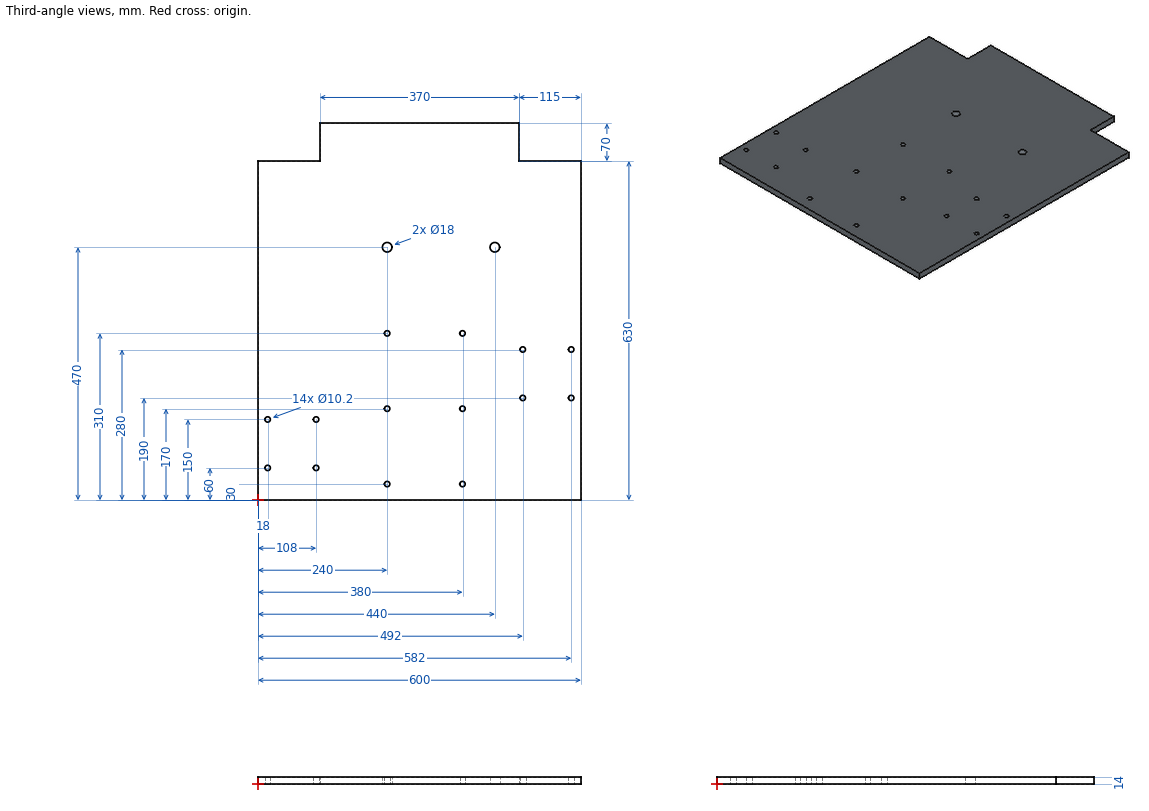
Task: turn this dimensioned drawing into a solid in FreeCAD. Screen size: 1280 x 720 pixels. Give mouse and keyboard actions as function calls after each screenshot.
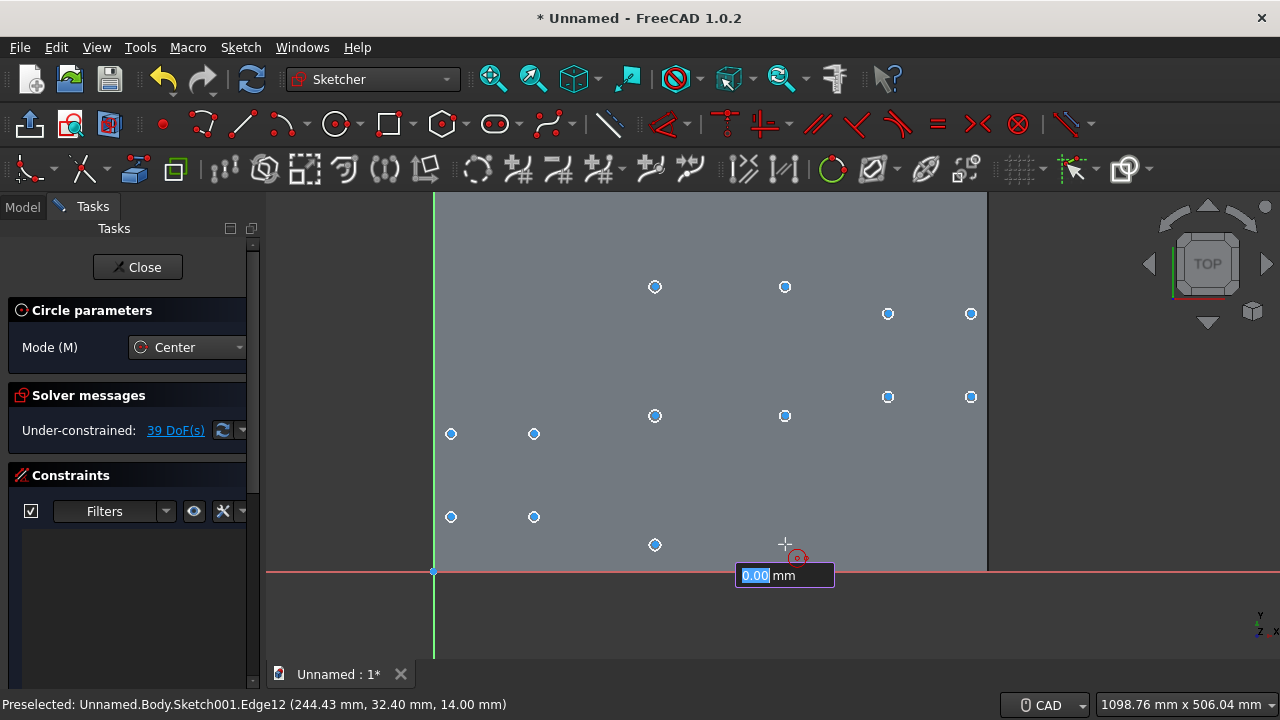
scroll(788, 541, up, 7)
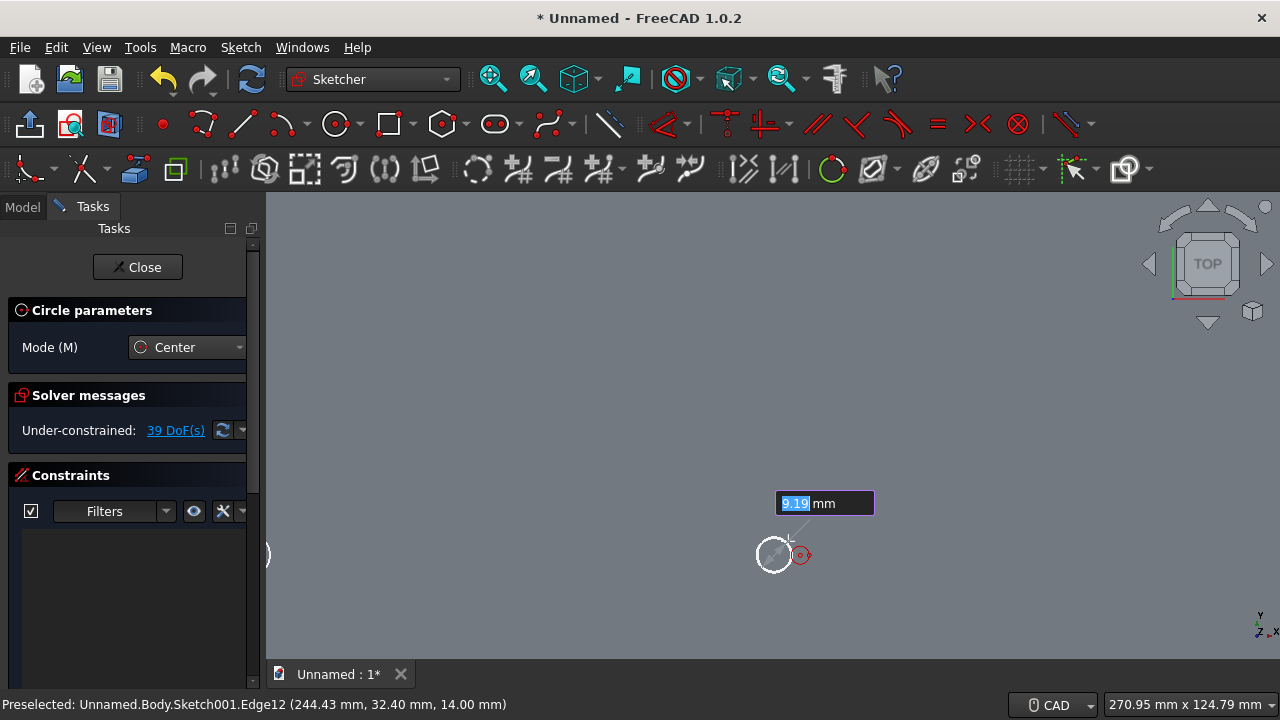
click(786, 537)
key(Escape)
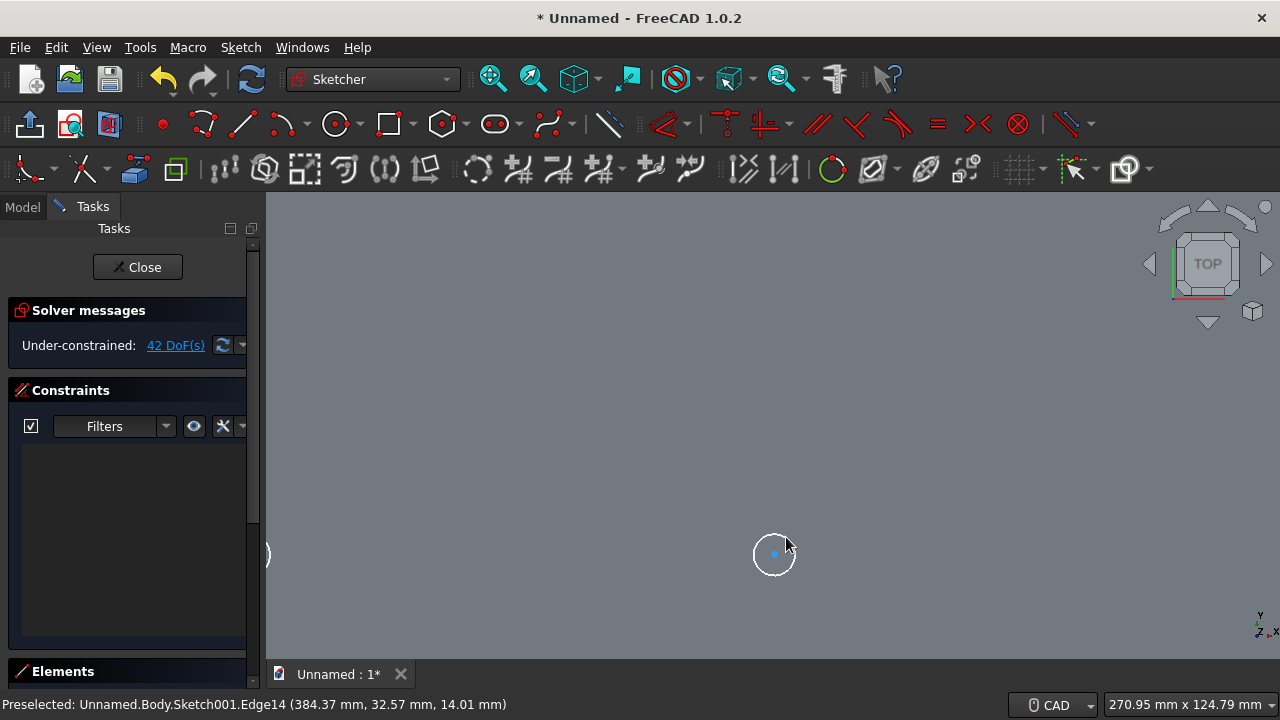
scroll(788, 541, down, 7)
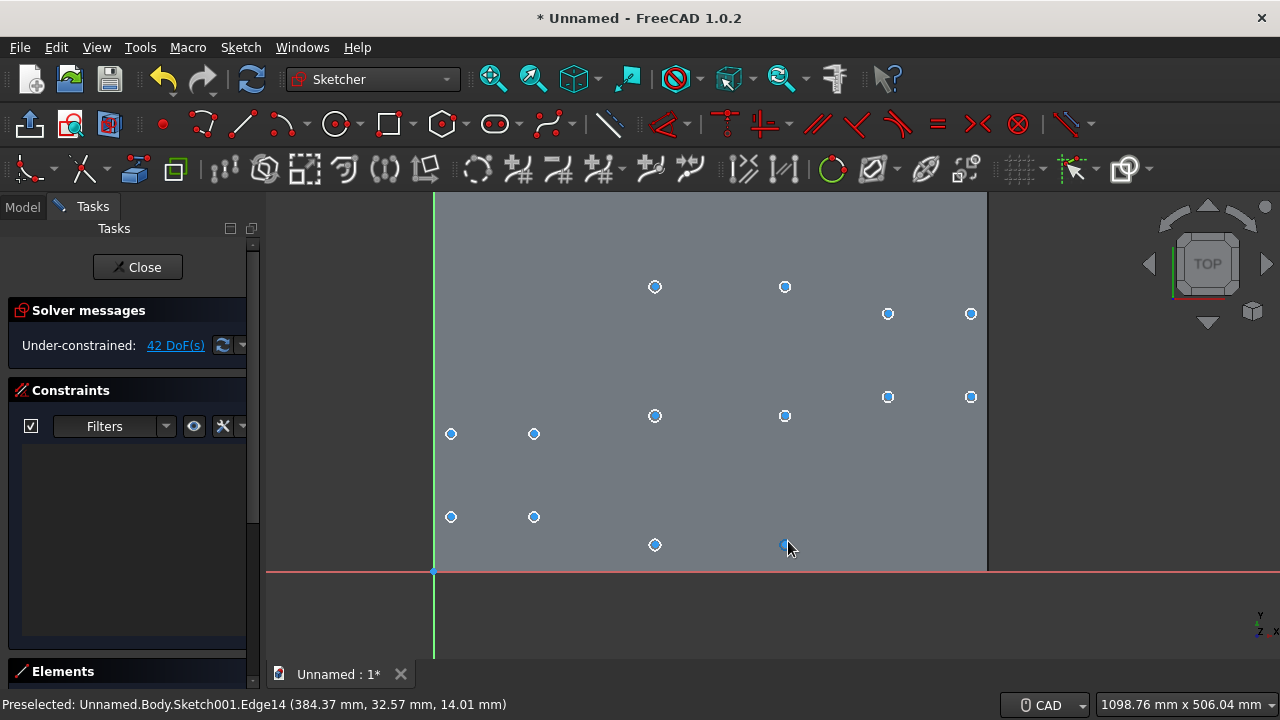
scroll(454, 431, up, 6)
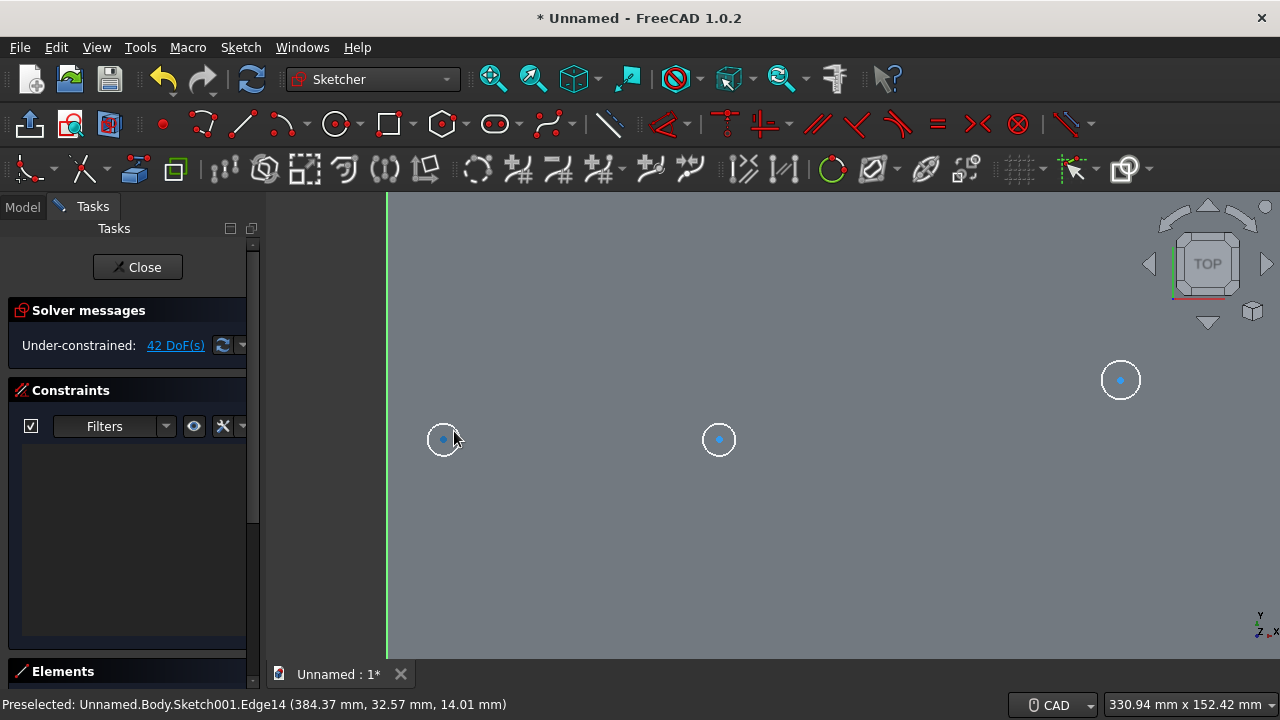
click(455, 428)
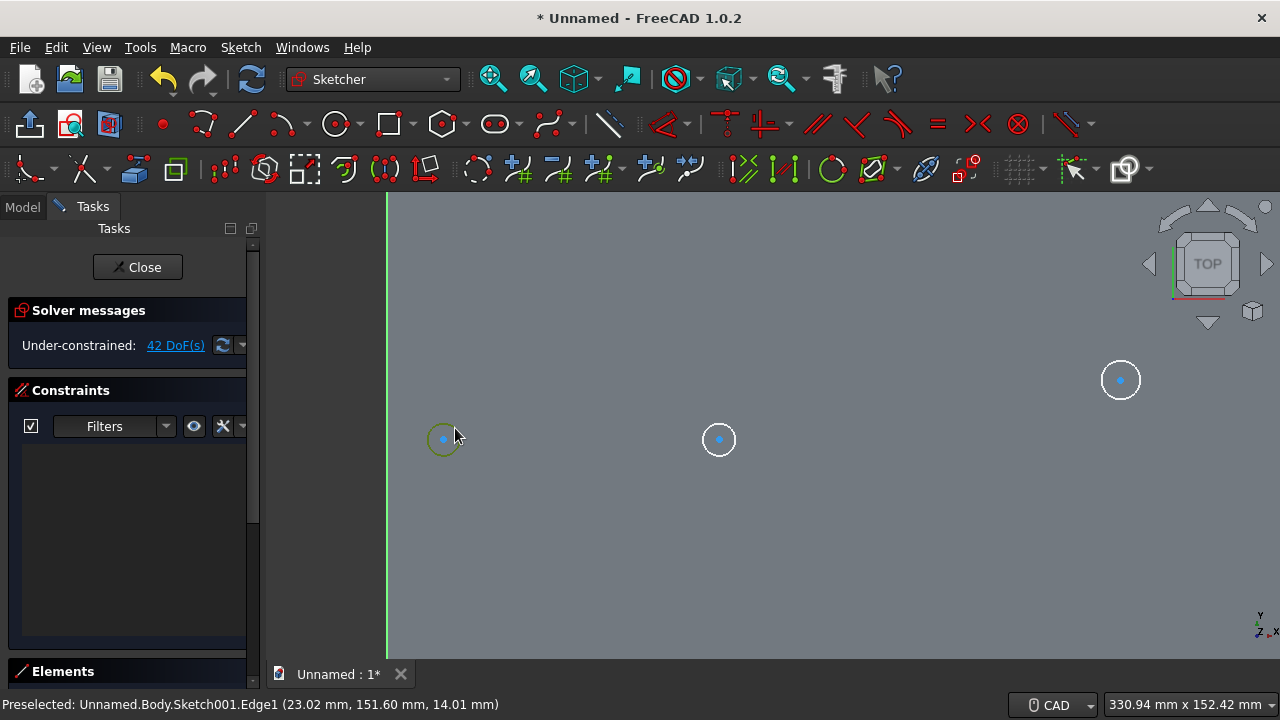
click(731, 428)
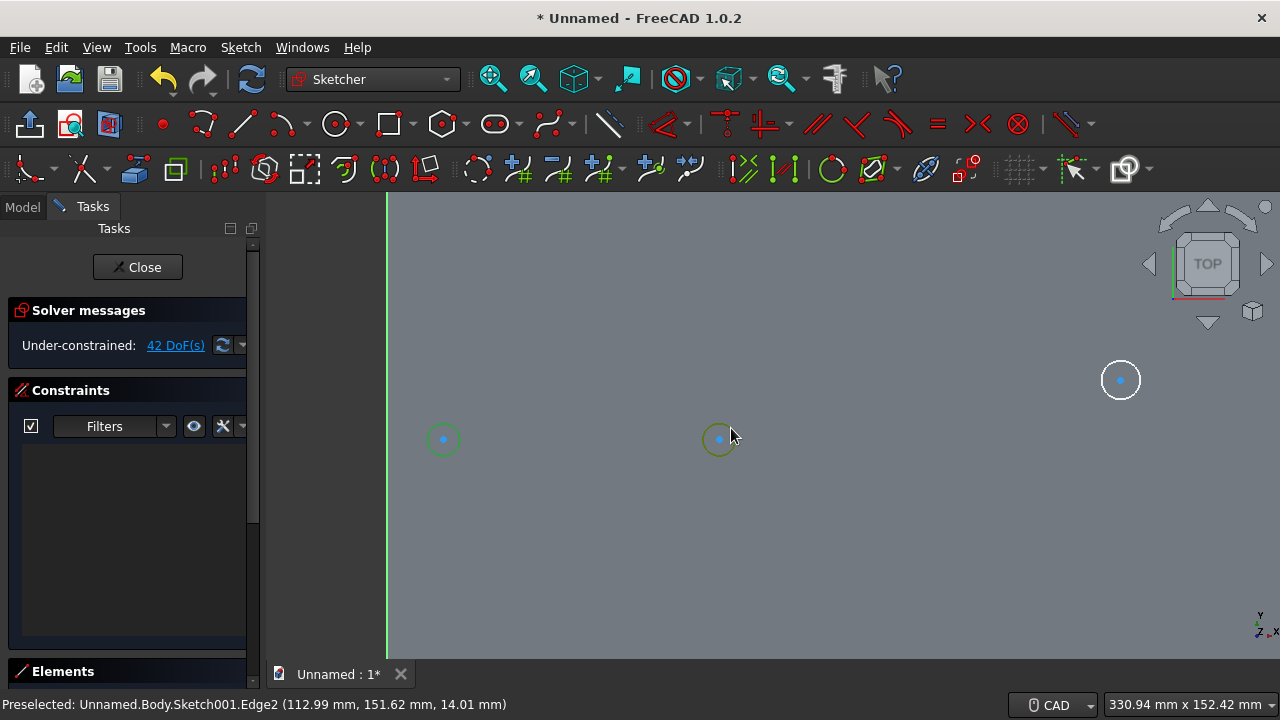
scroll(454, 431, down, 6)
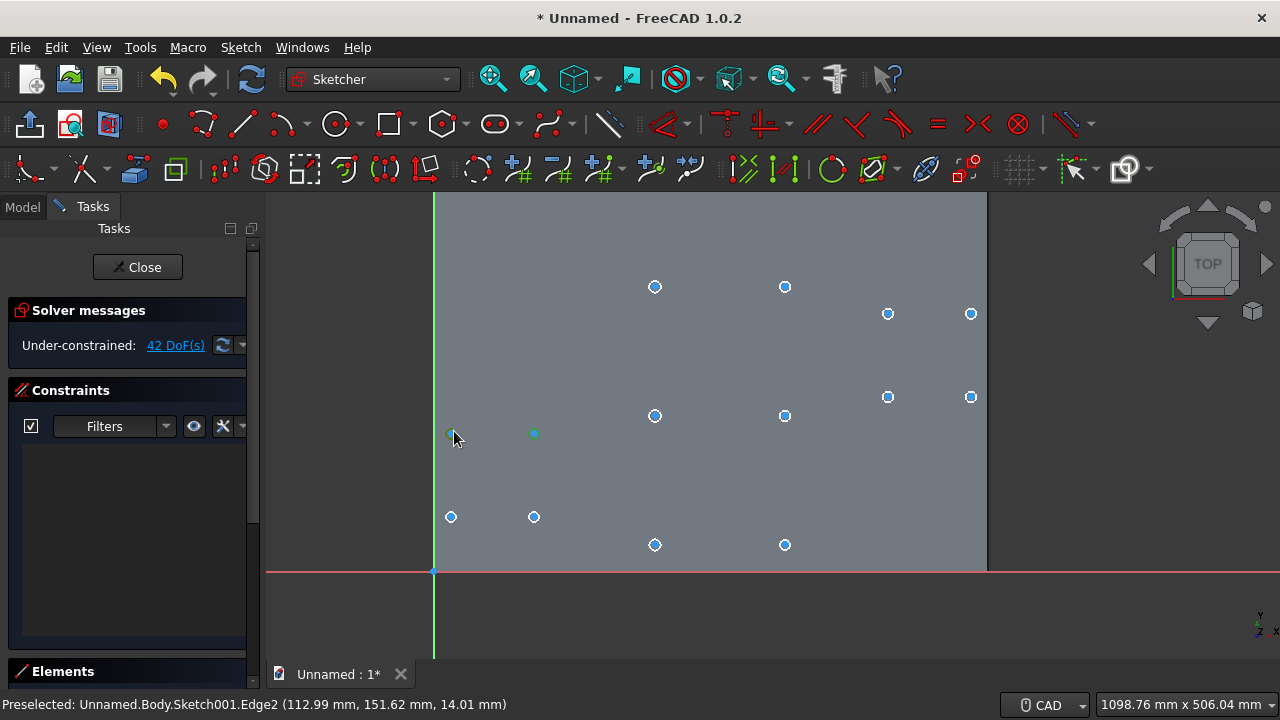
scroll(454, 514, up, 6)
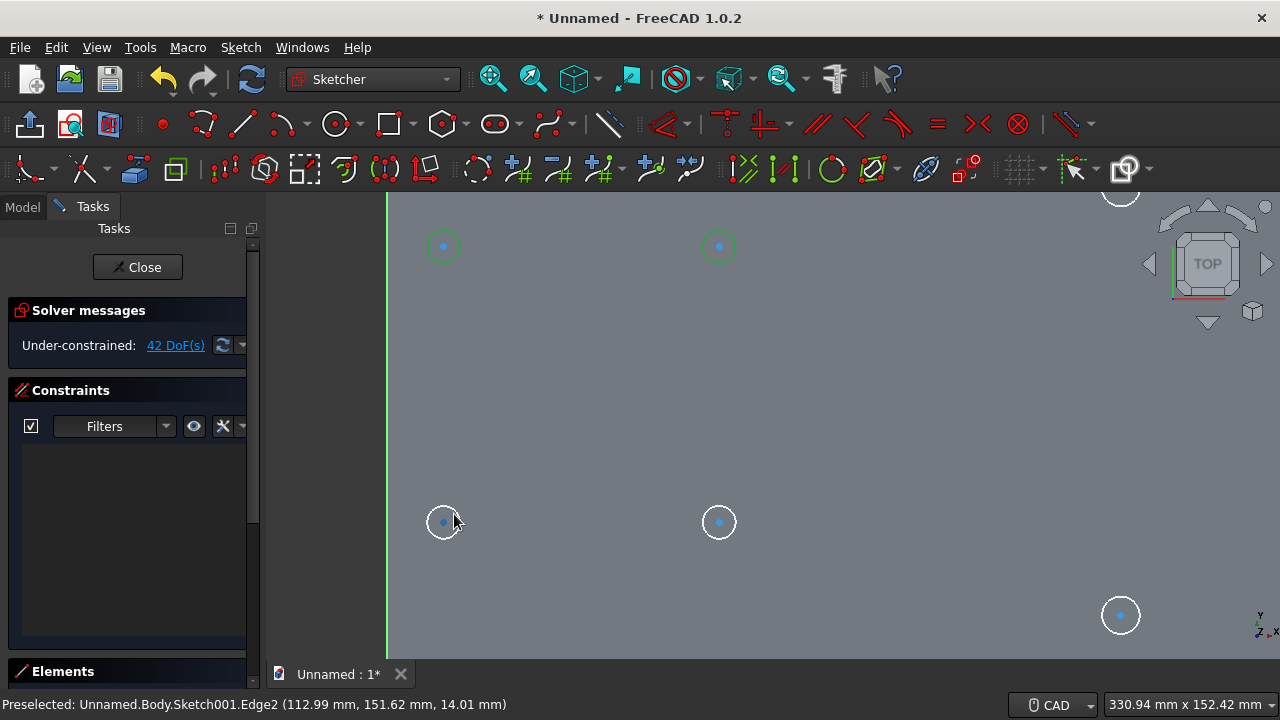
click(455, 511)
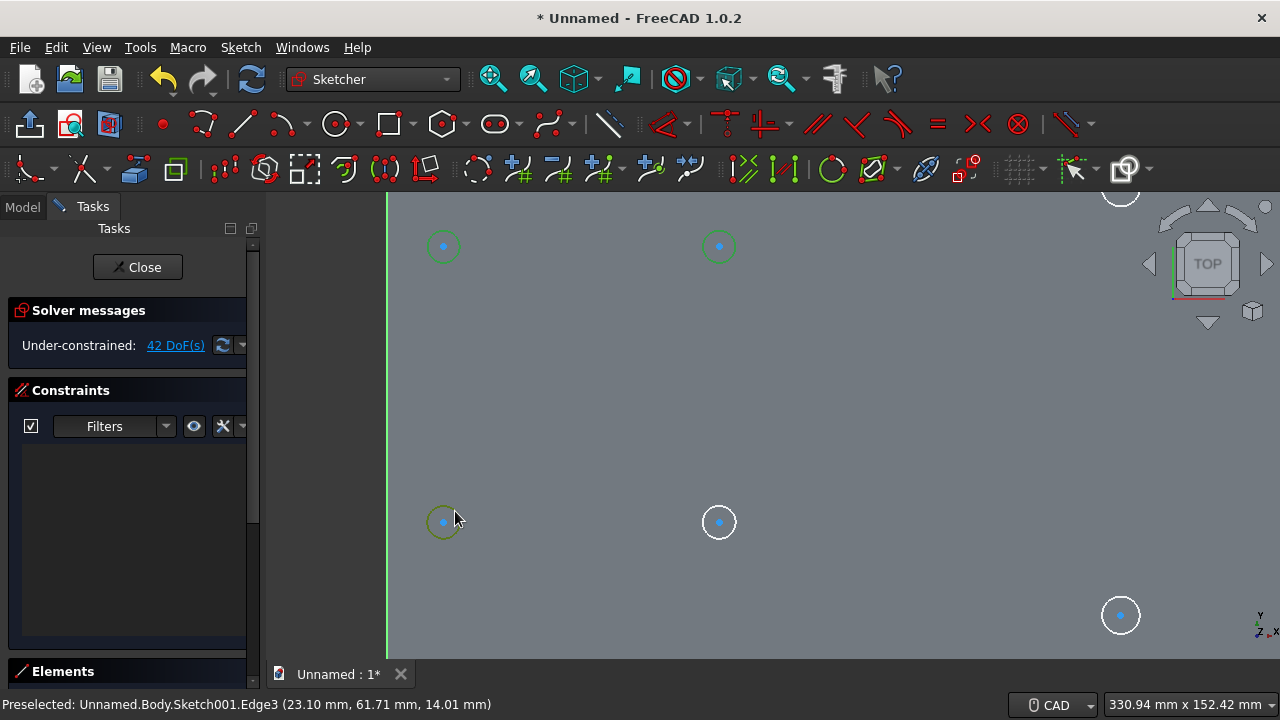
click(731, 511)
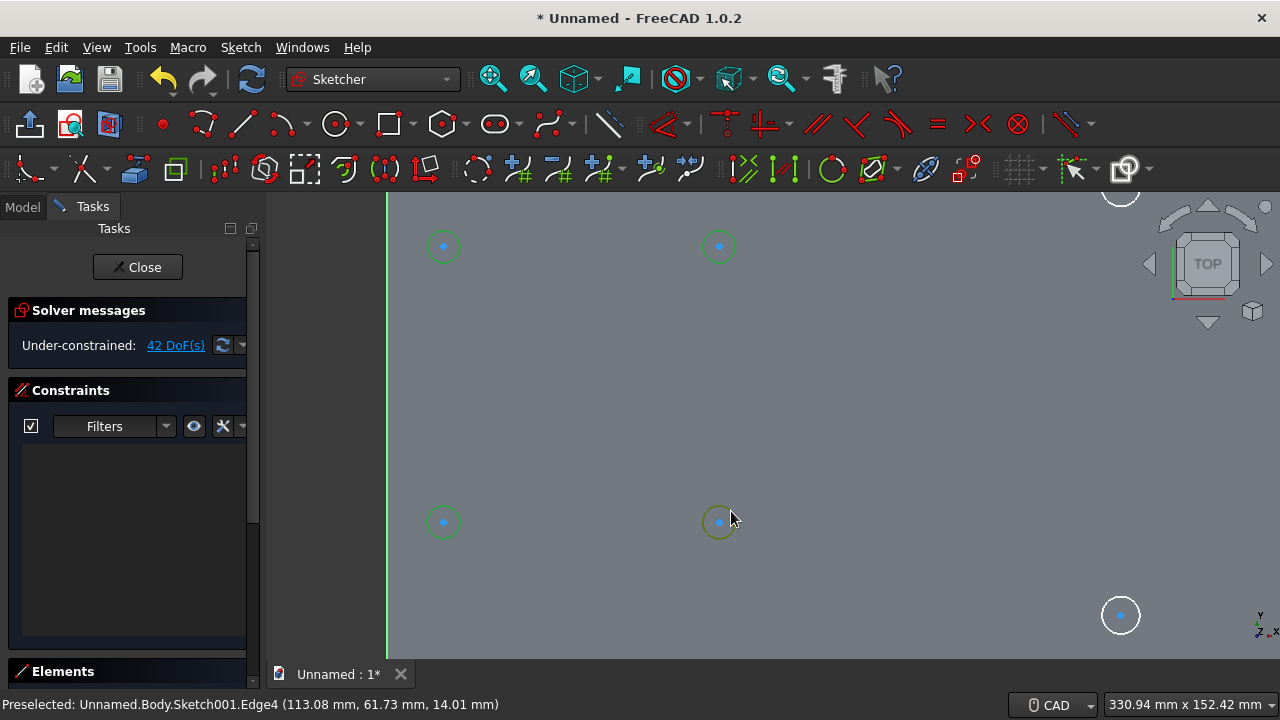
scroll(454, 514, down, 6)